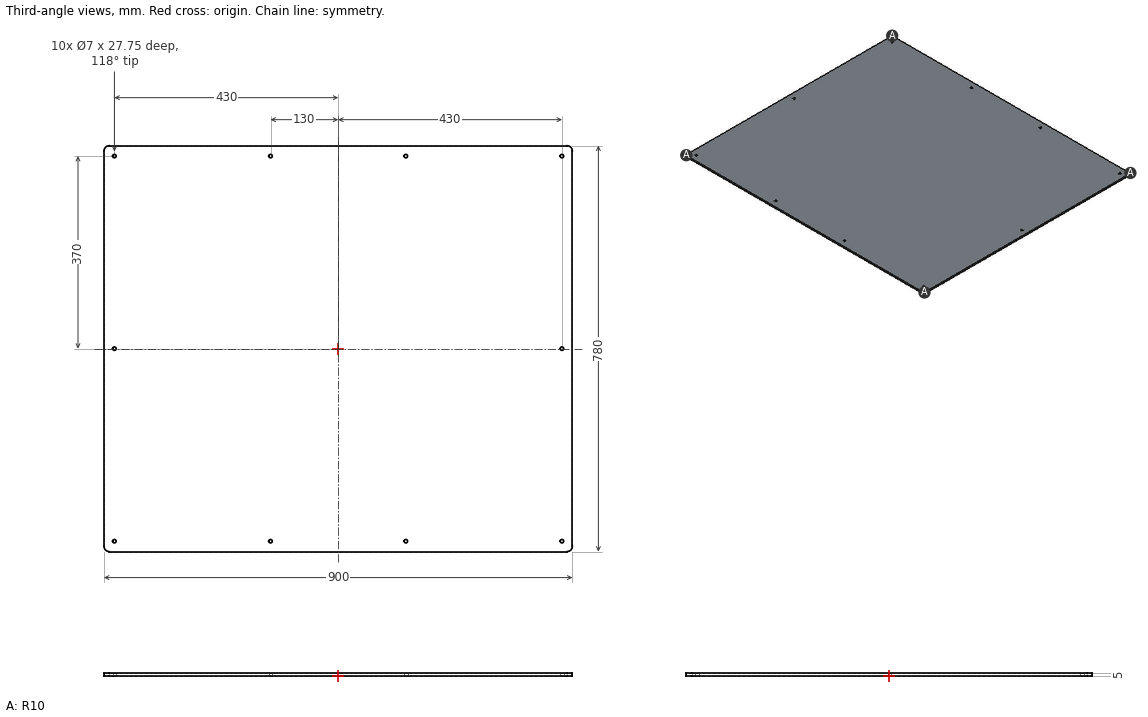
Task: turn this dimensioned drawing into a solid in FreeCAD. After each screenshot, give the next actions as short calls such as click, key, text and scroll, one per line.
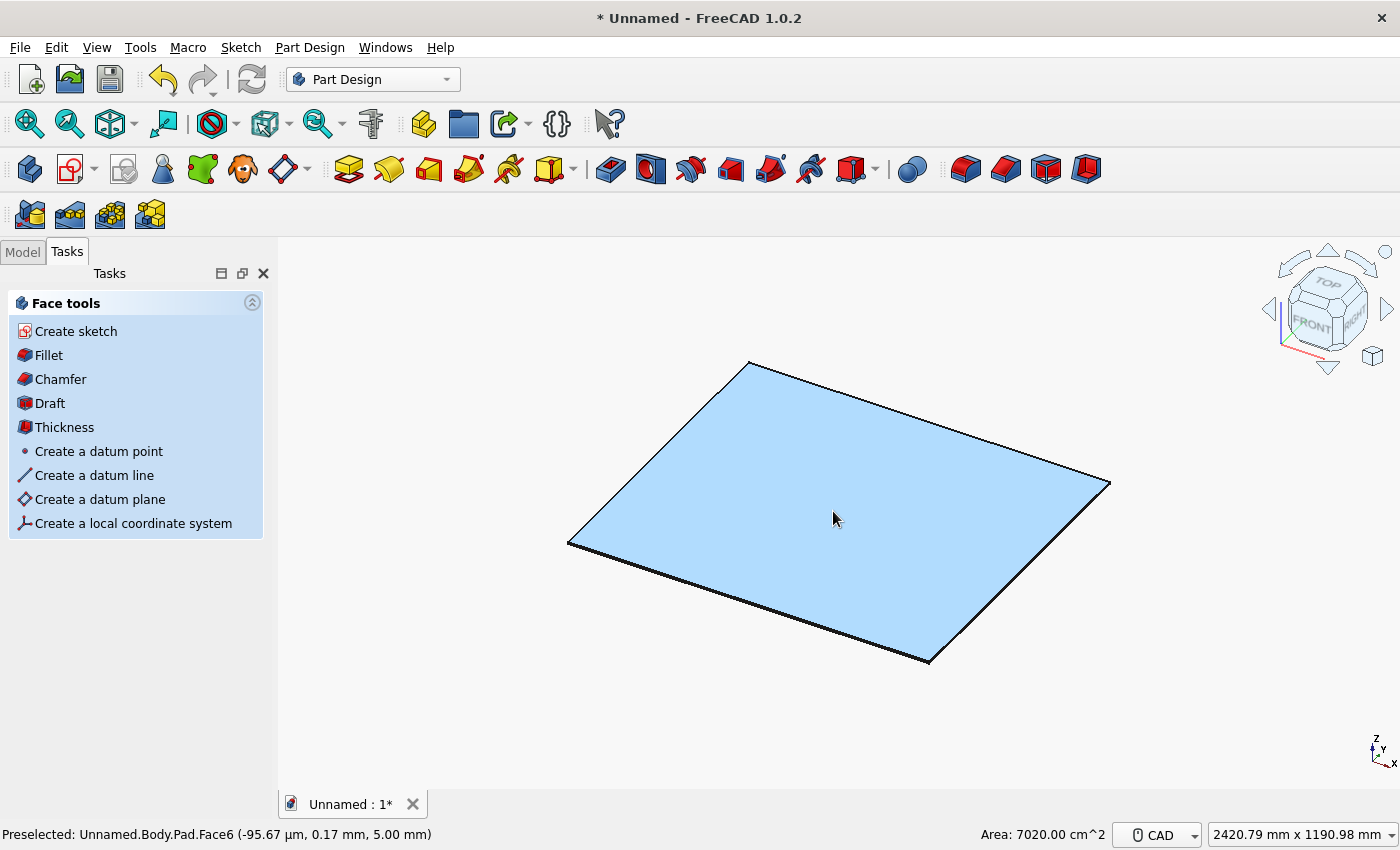
click(70, 170)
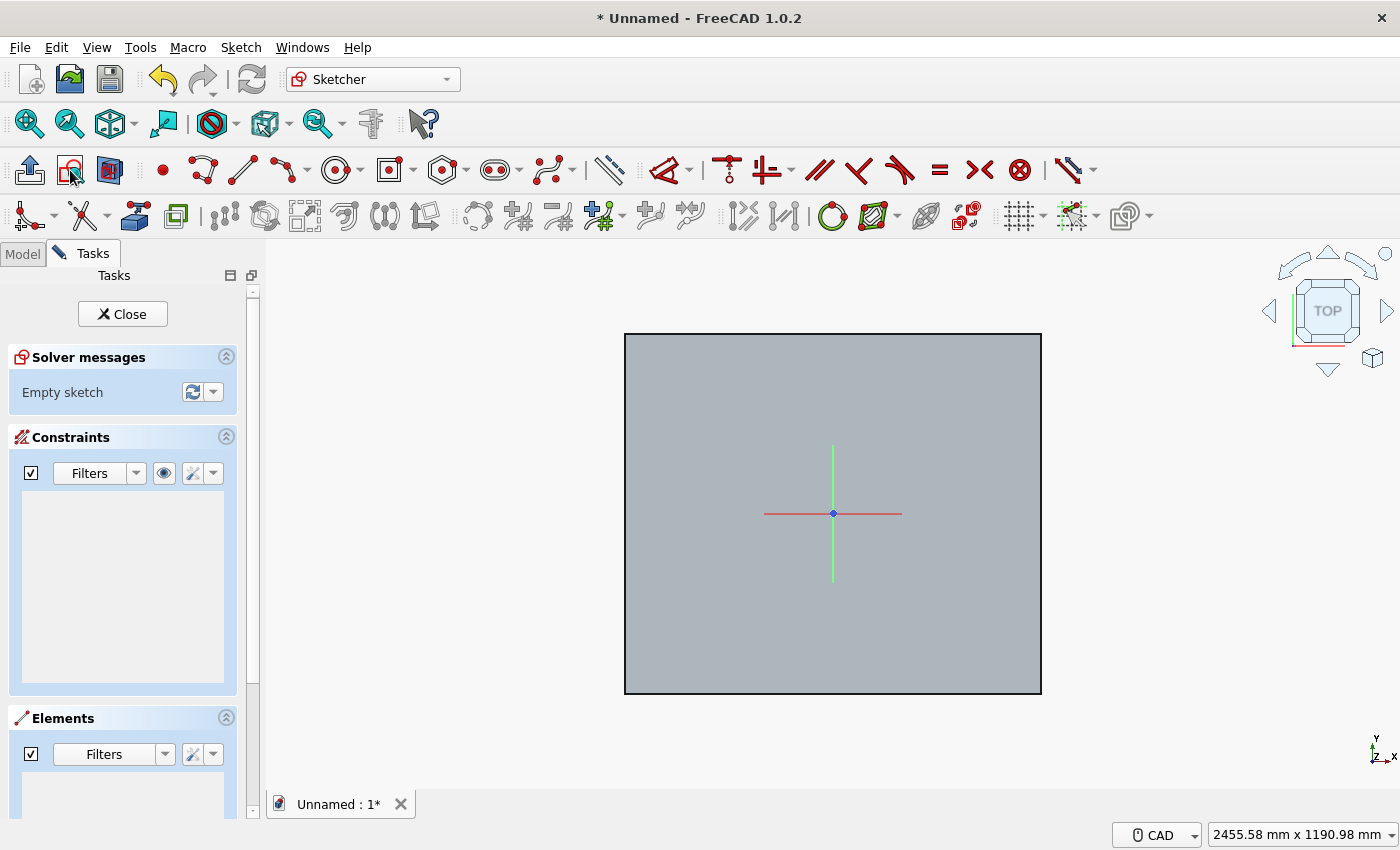
click(336, 170)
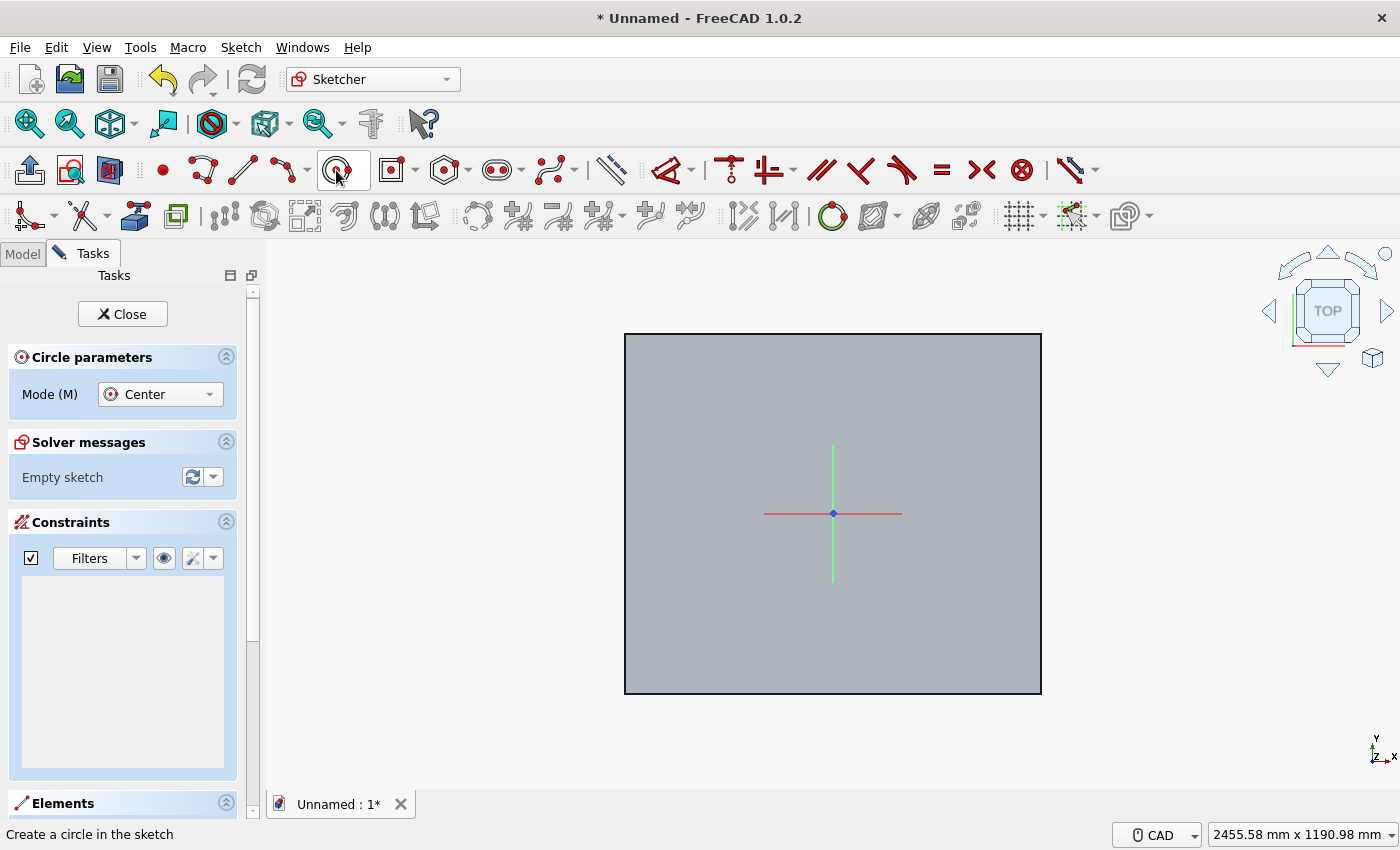
scroll(634, 343, up, 14)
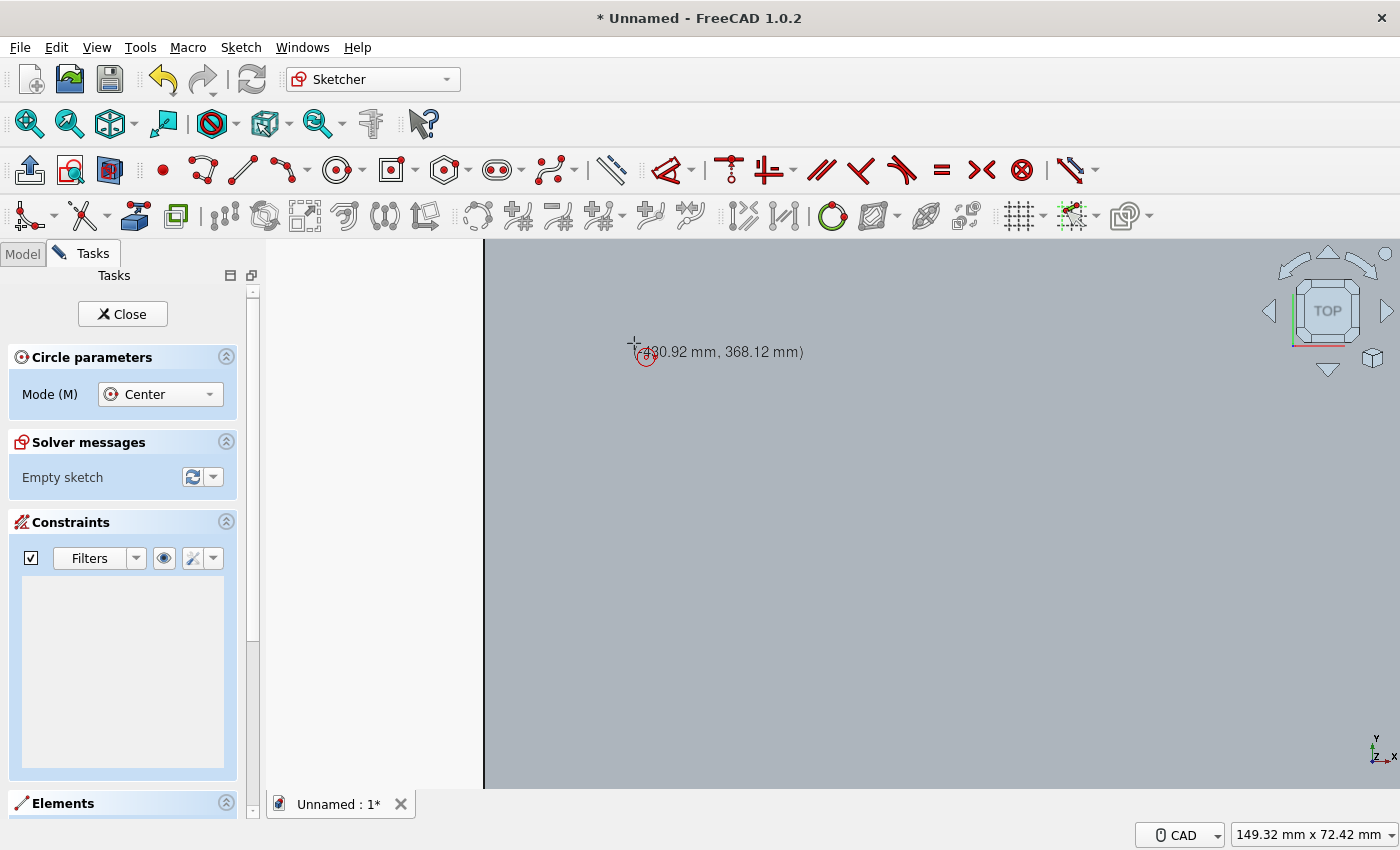
scroll(561, 343, down, 14)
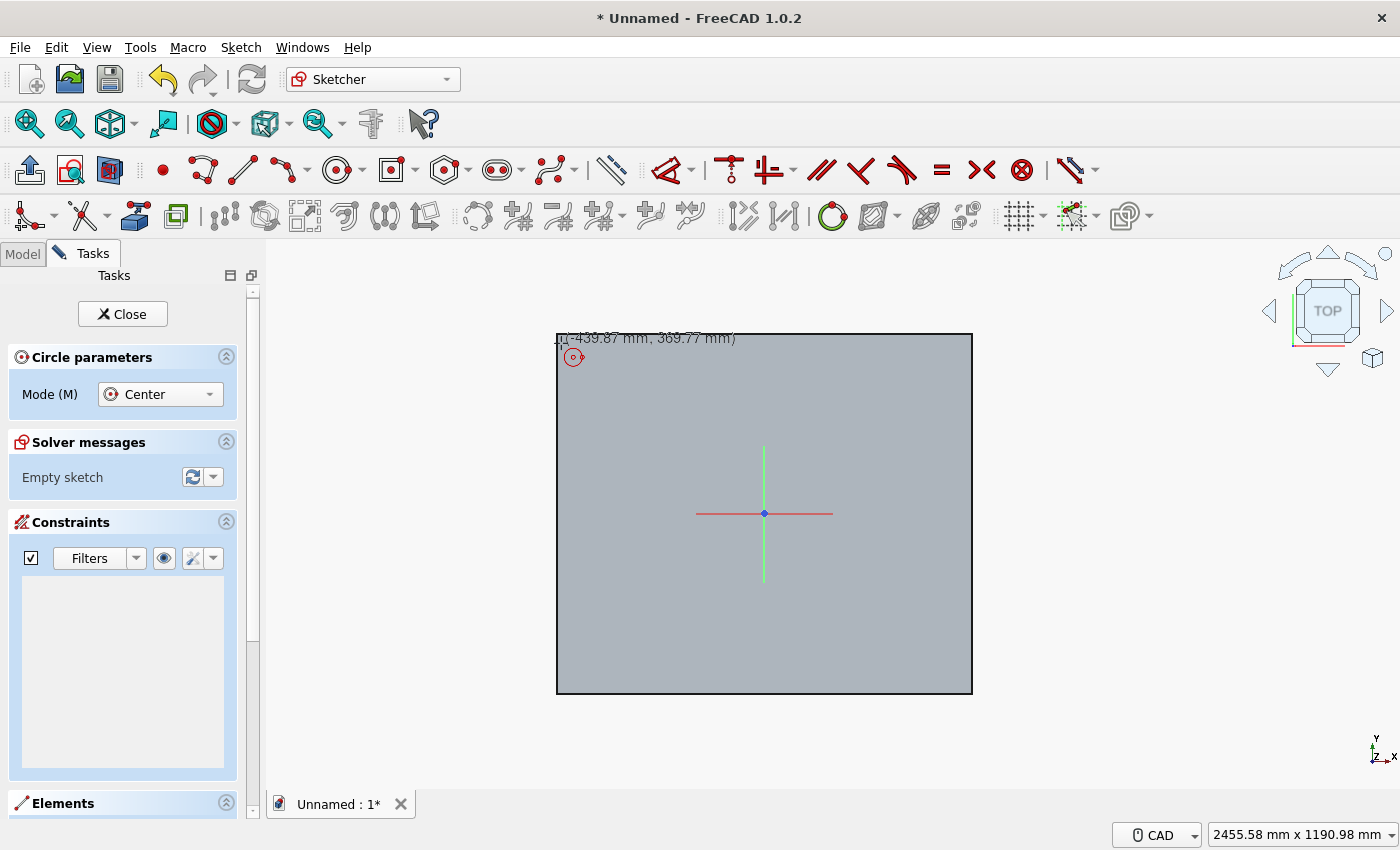
click(566, 343)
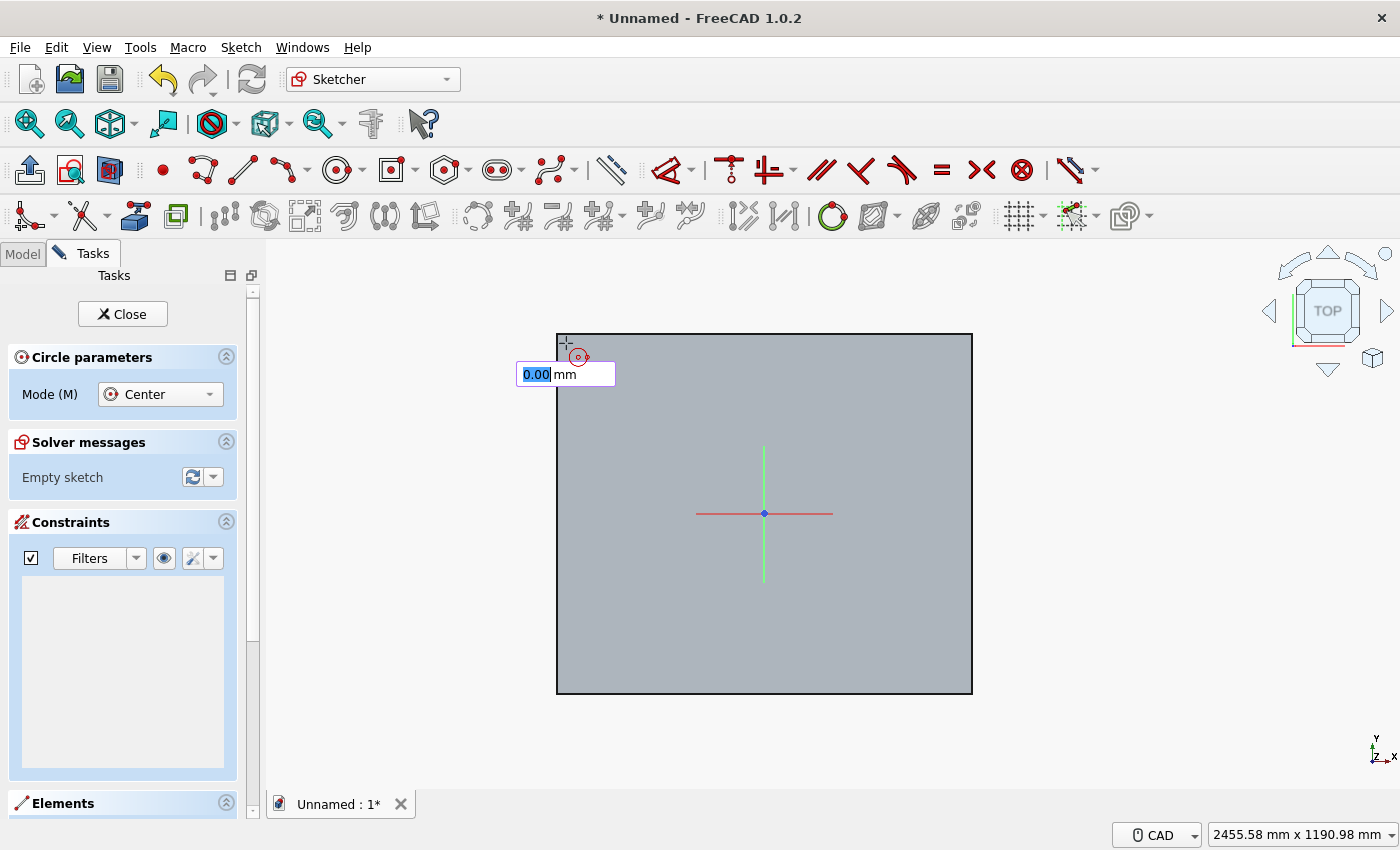
scroll(567, 342, up, 12)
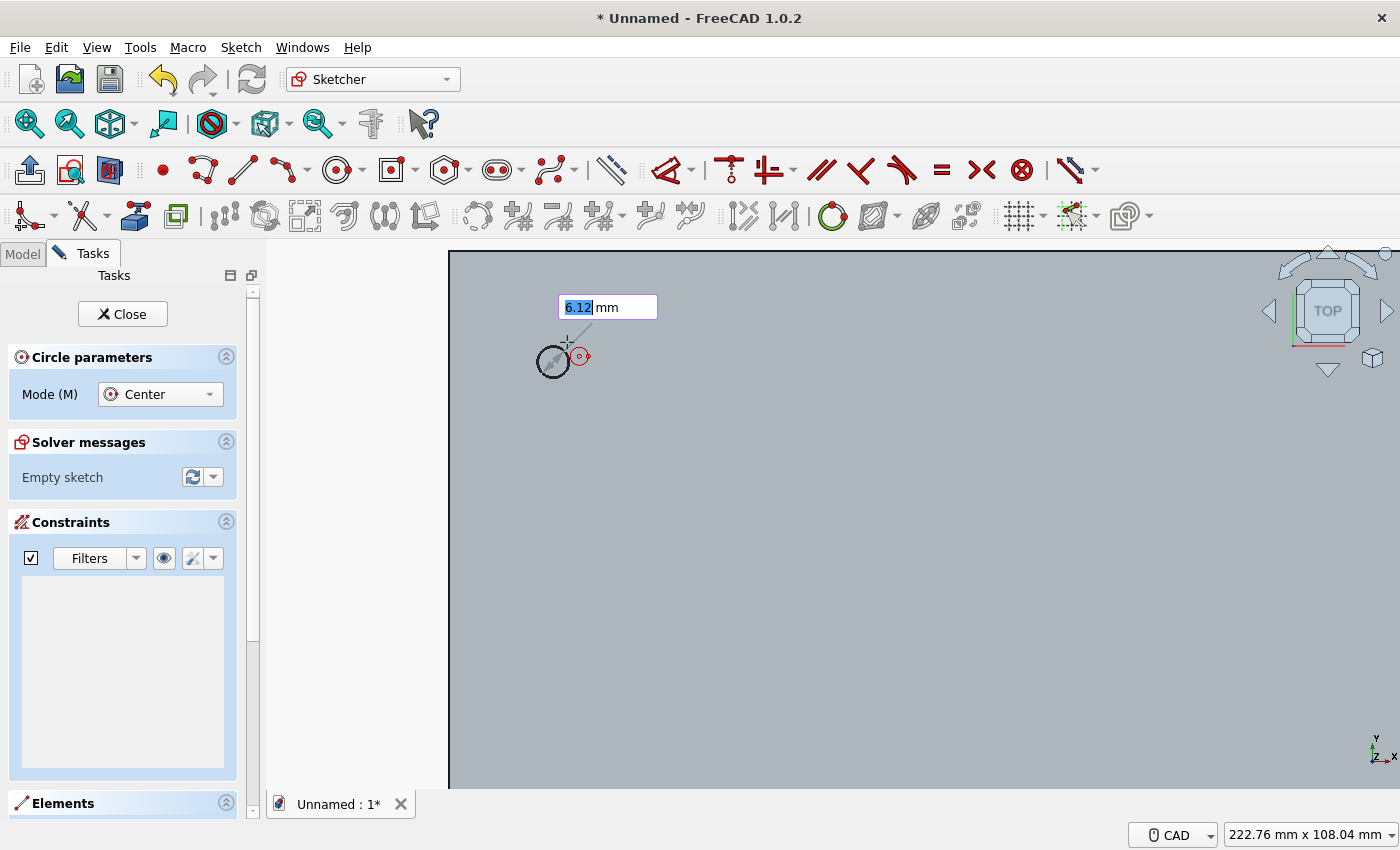
click(564, 340)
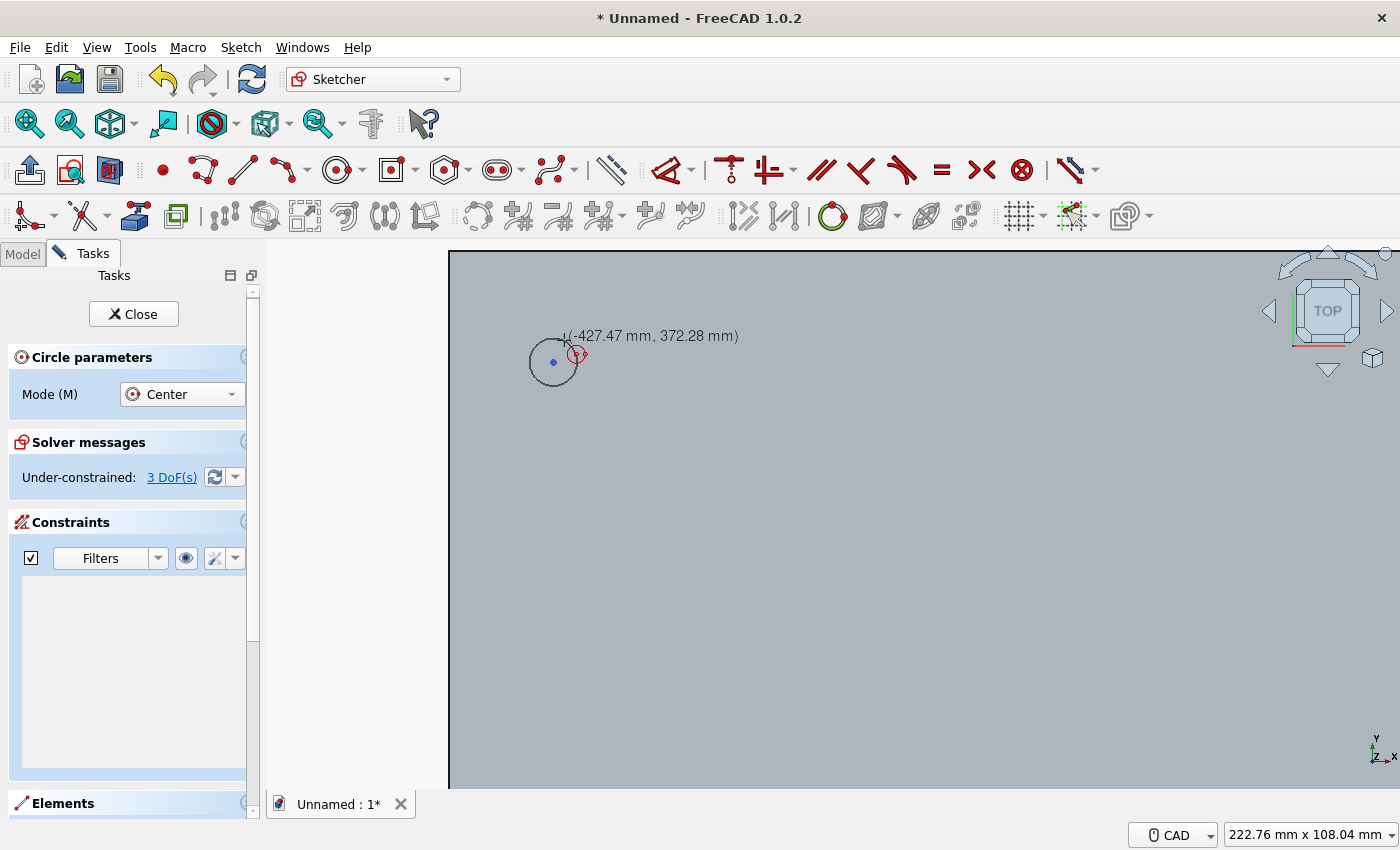
scroll(567, 342, down, 12)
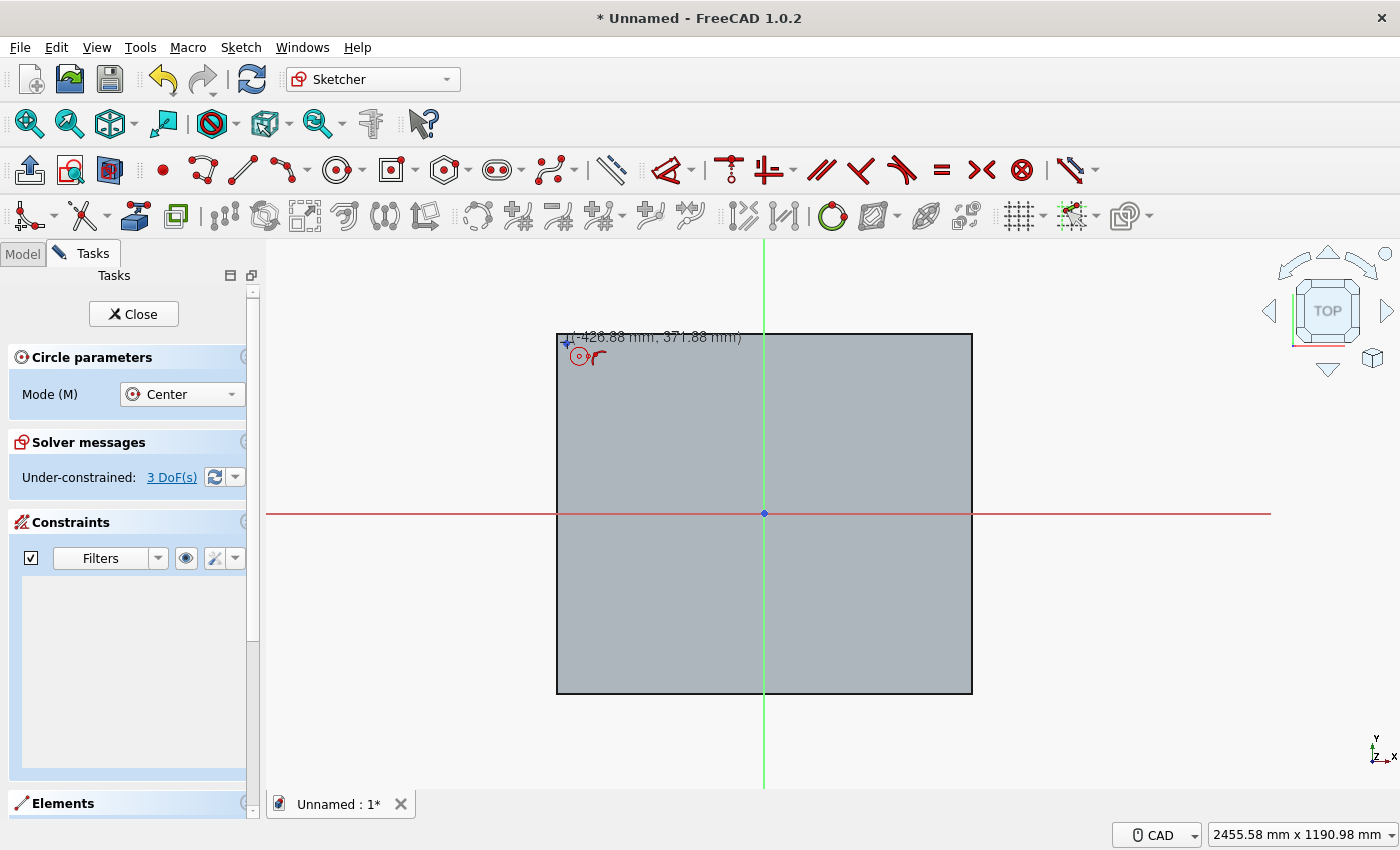
scroll(963, 343, up, 14)